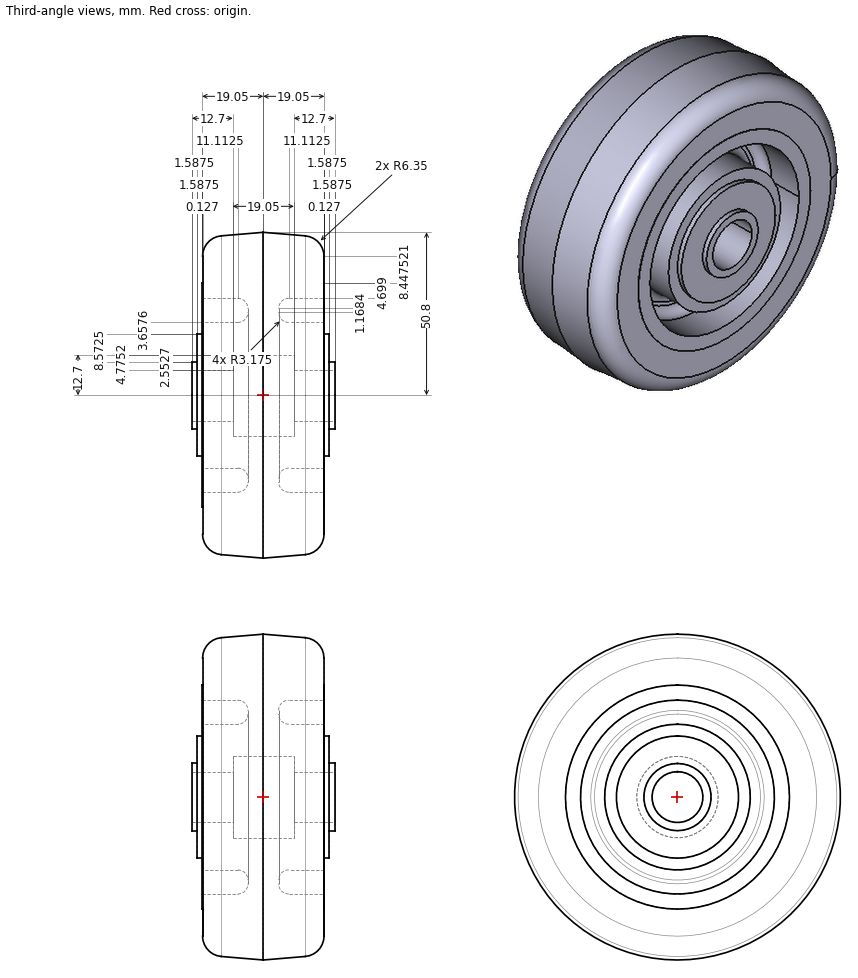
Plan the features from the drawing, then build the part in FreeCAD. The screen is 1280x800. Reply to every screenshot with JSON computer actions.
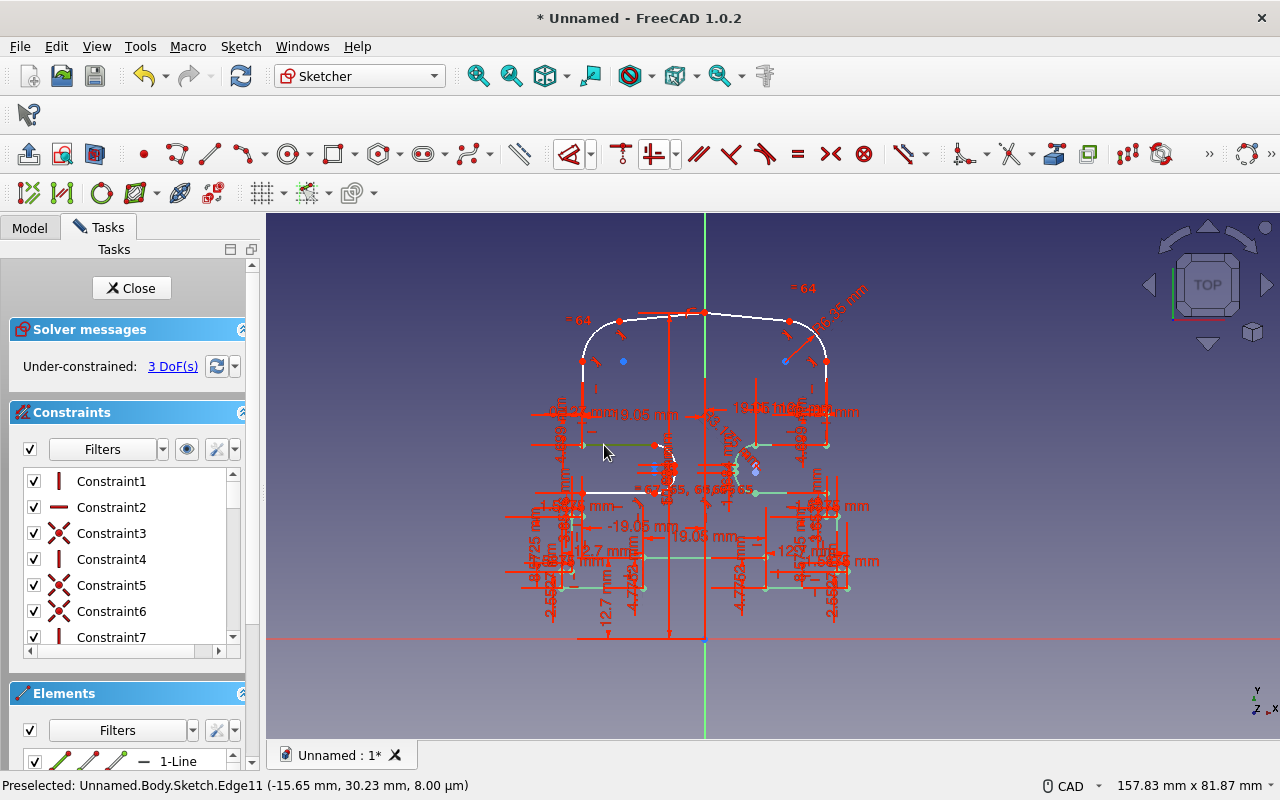
{"action": "left_click", "coordinate": [590, 154]}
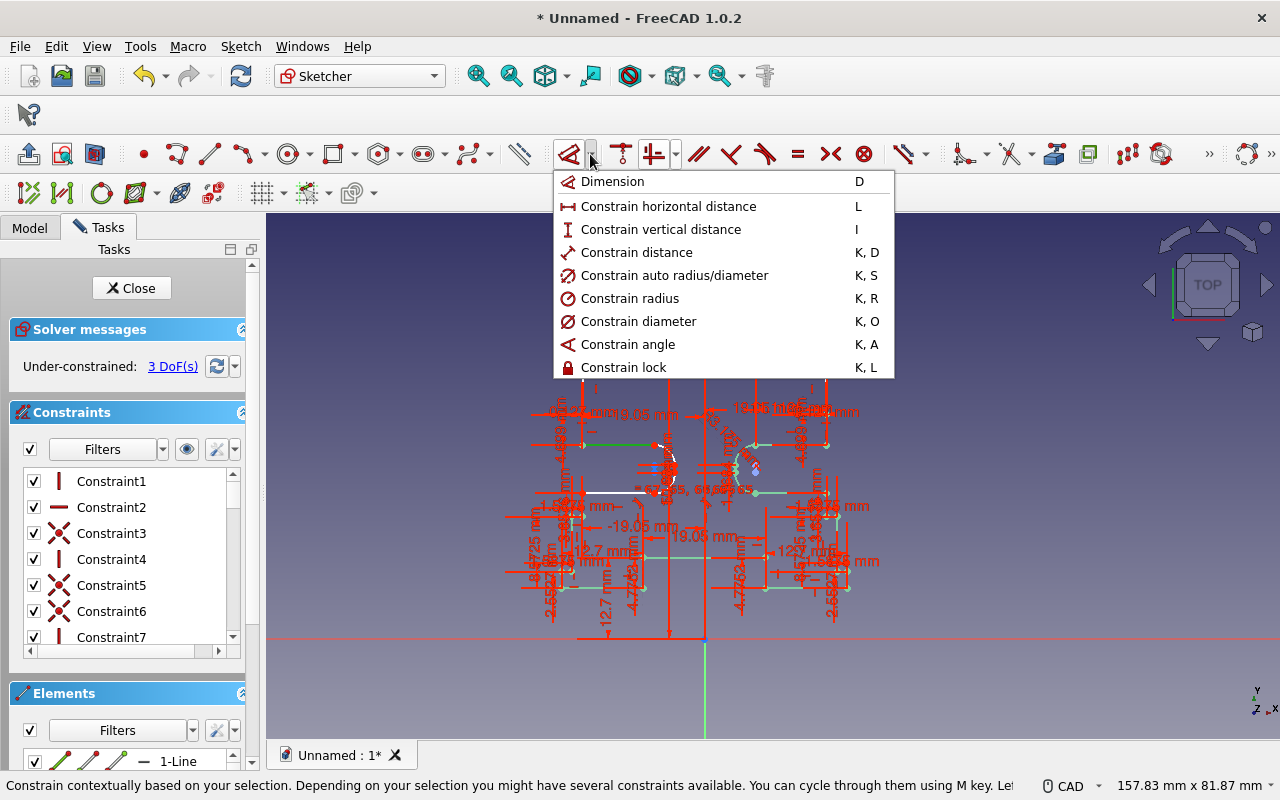
{"action": "left_click", "coordinate": [724, 206]}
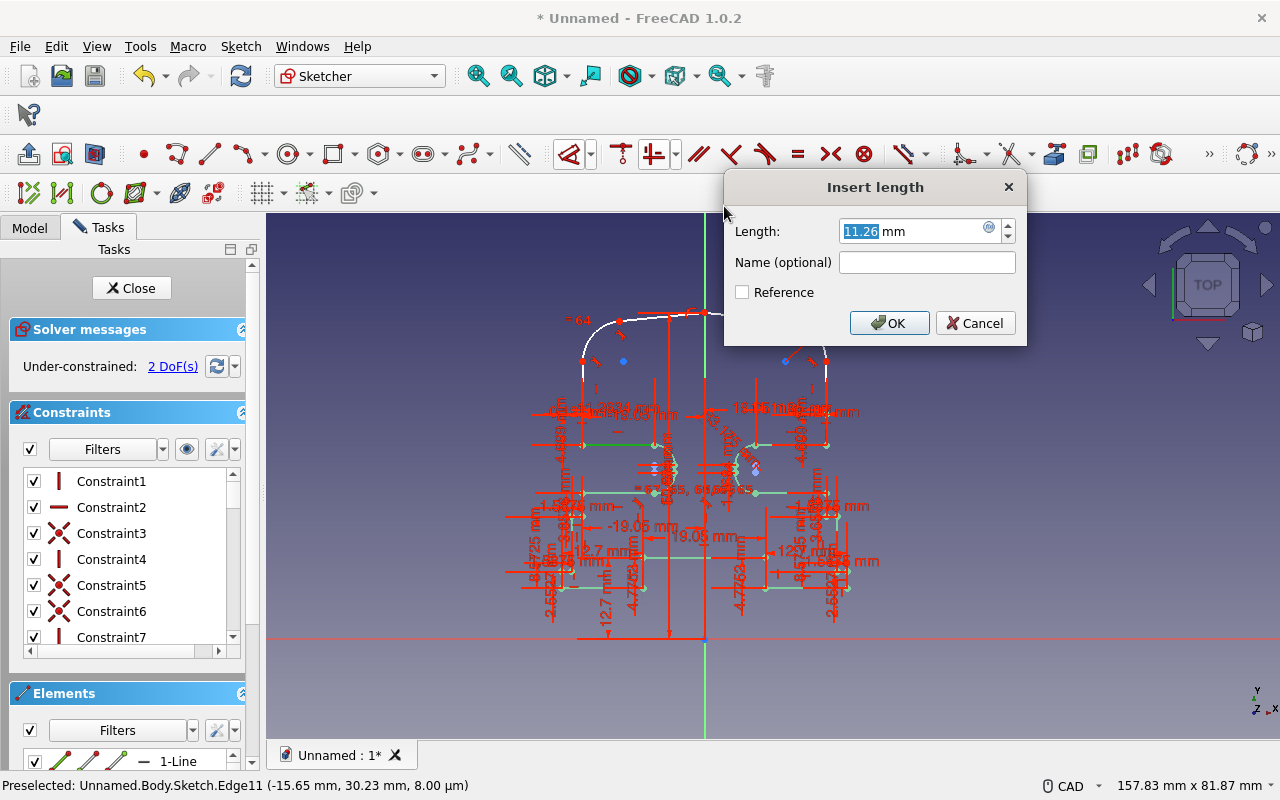
{"action": "type", "text": "11.1125"}
{"action": "key", "text": "Return"}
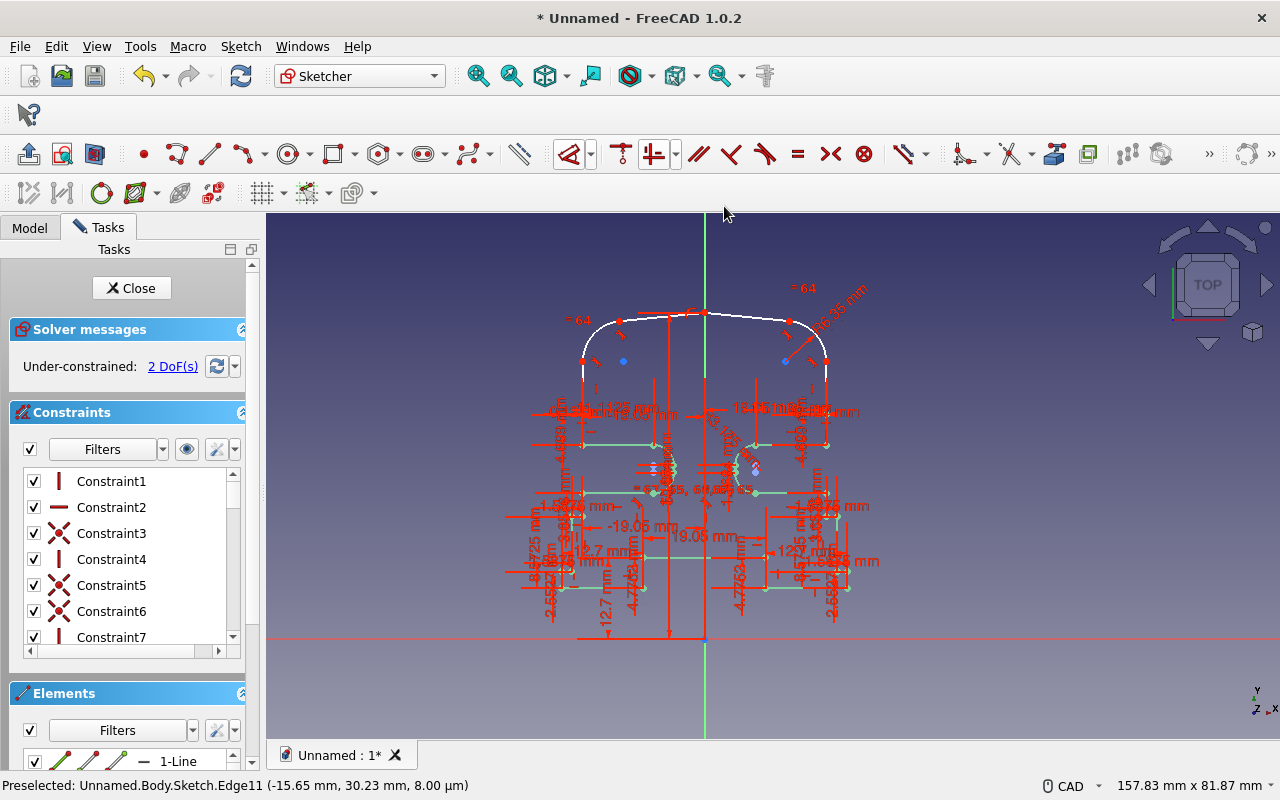
{"action": "left_click", "coordinate": [826, 399]}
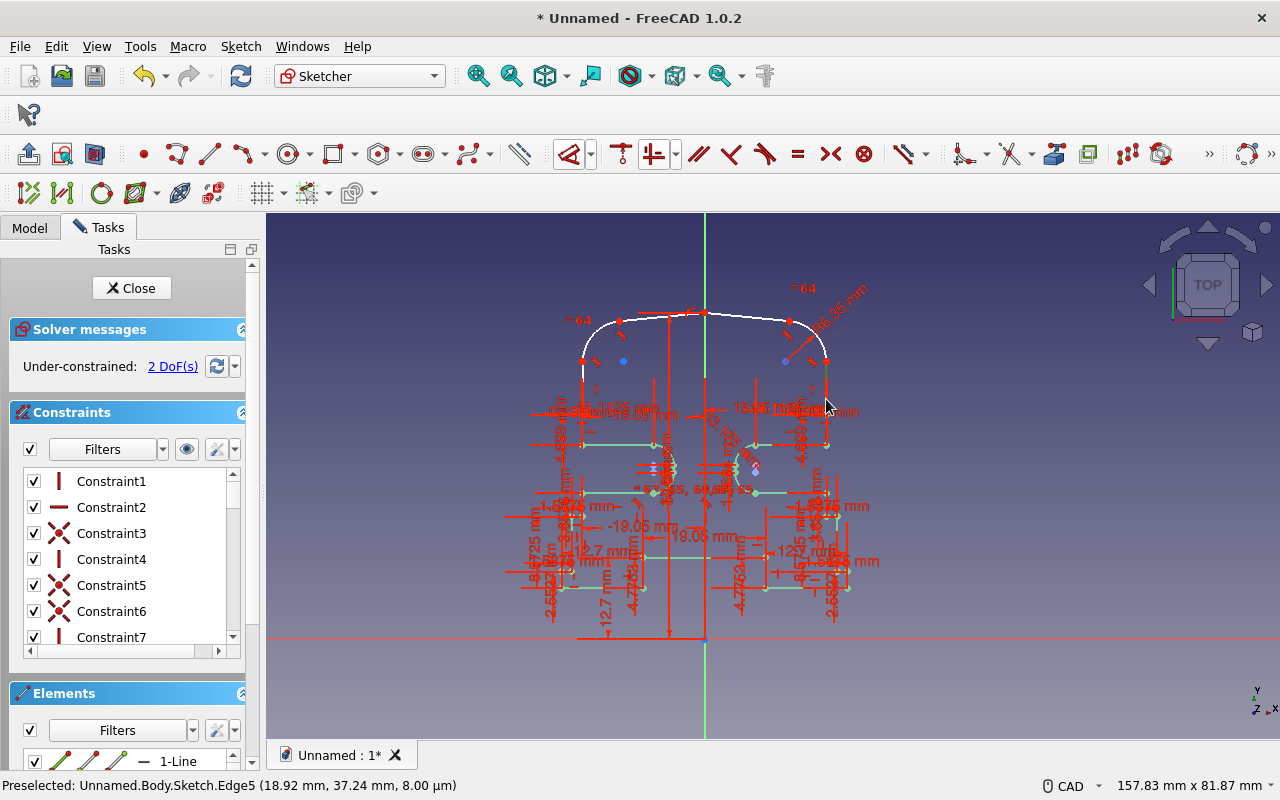
{"action": "left_click", "coordinate": [590, 154]}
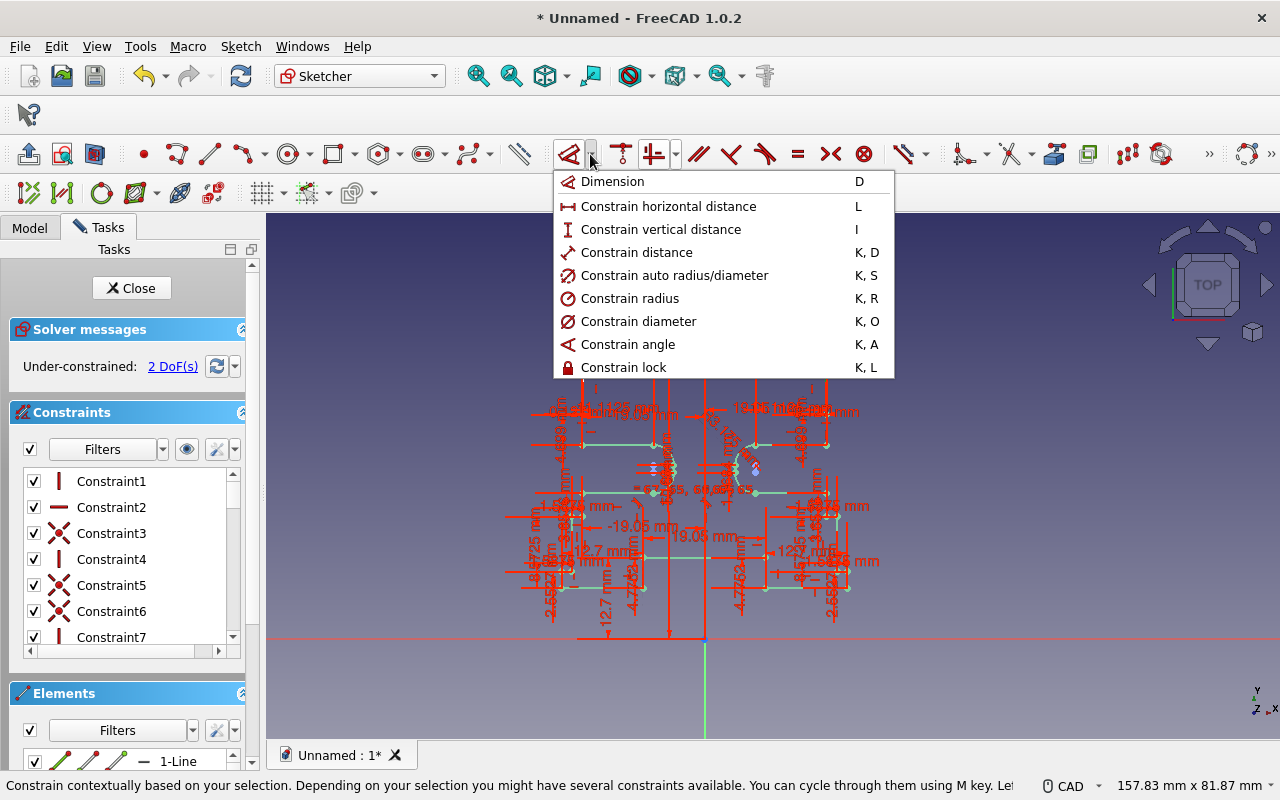
{"action": "left_click", "coordinate": [724, 230]}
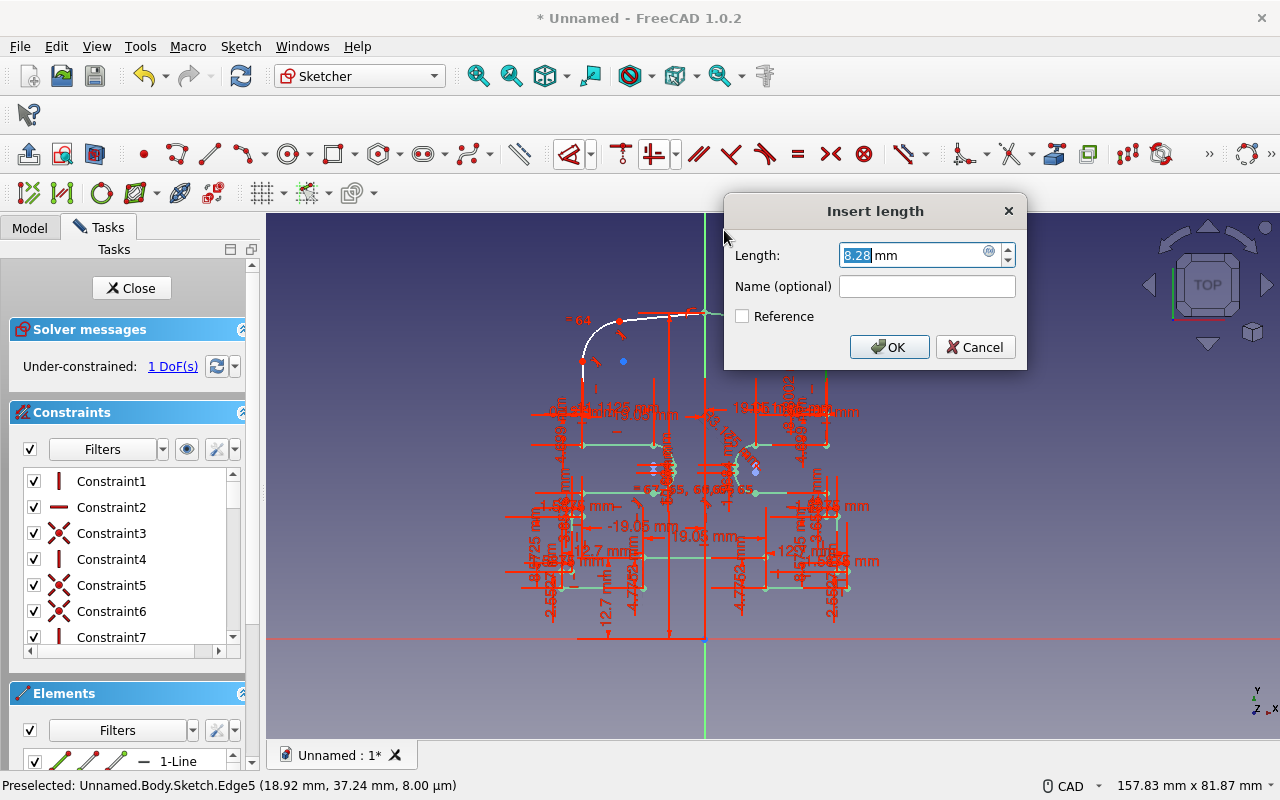
{"action": "type", "text": "8.447521"}
{"action": "key", "text": "Return"}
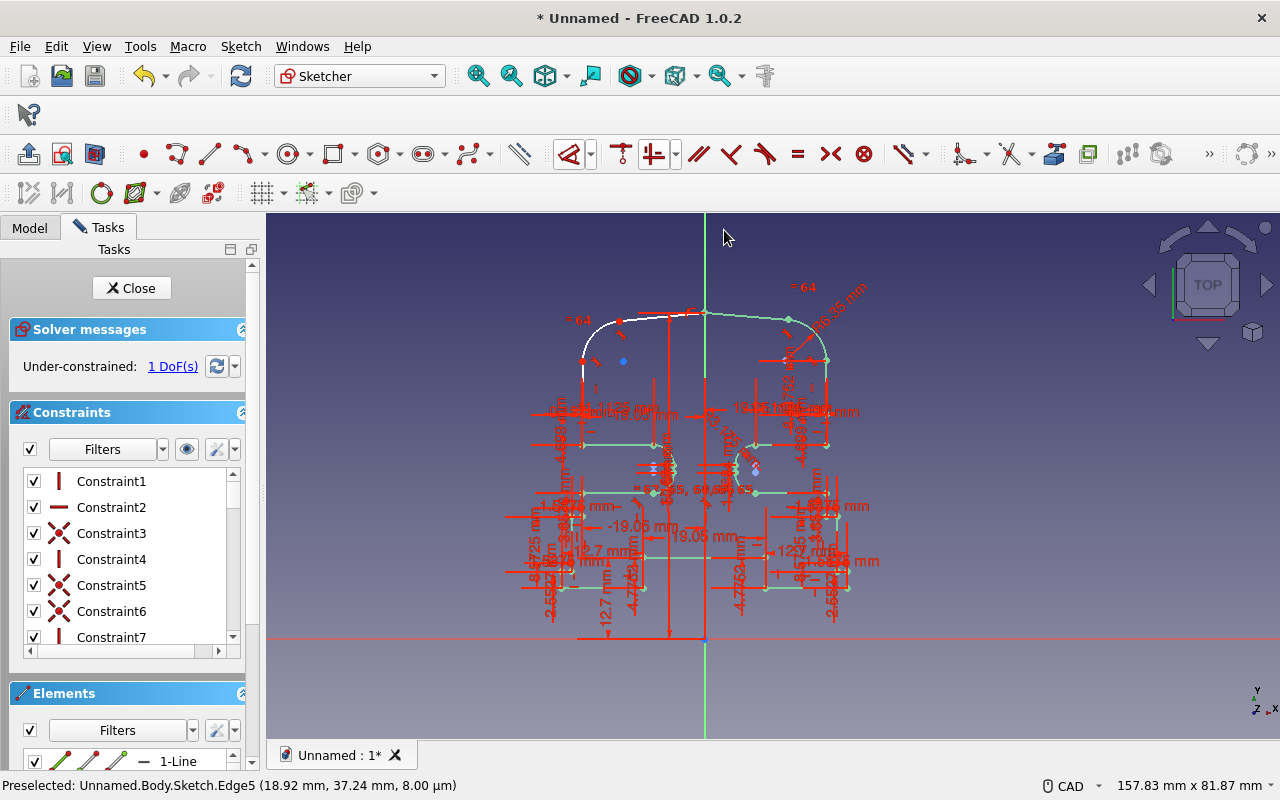
{"action": "left_click", "coordinate": [583, 378]}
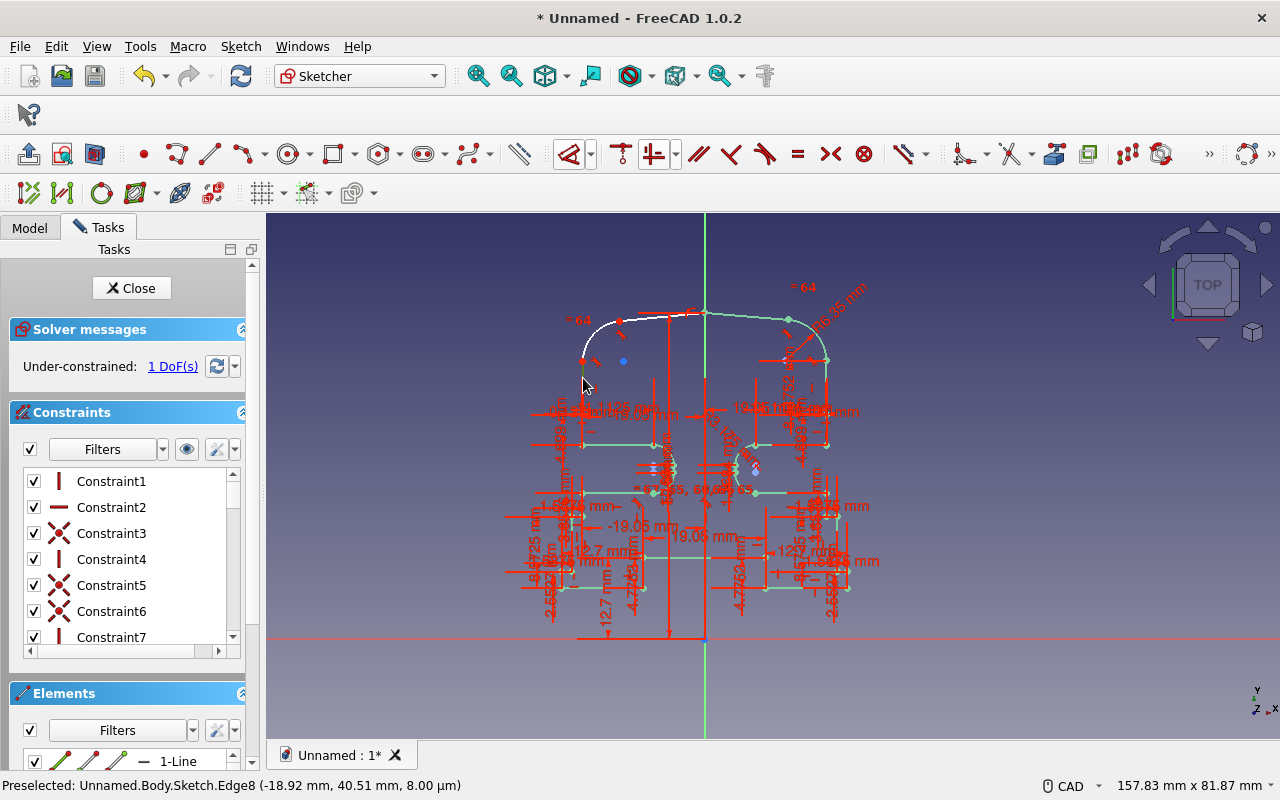
{"action": "key", "text": "i"}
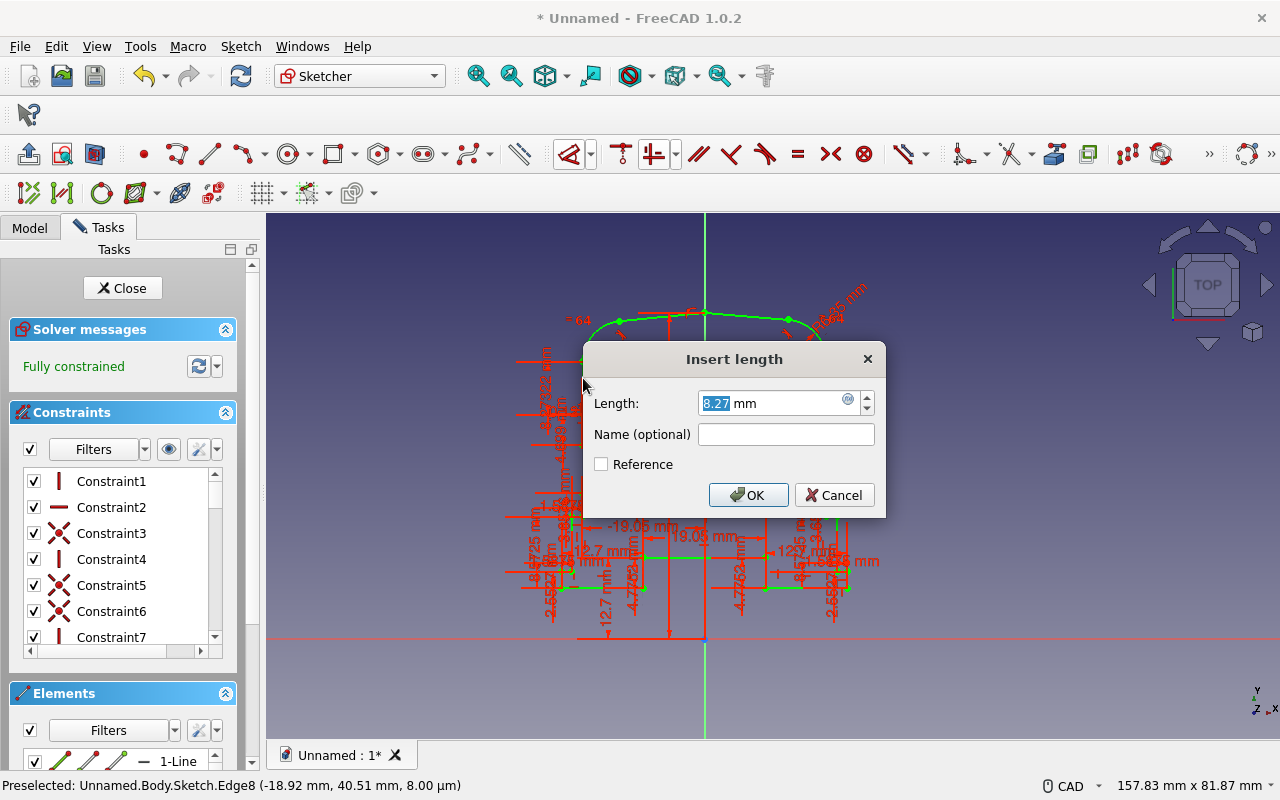
{"action": "type", "text": "8.447521"}
{"action": "key", "text": "Return"}